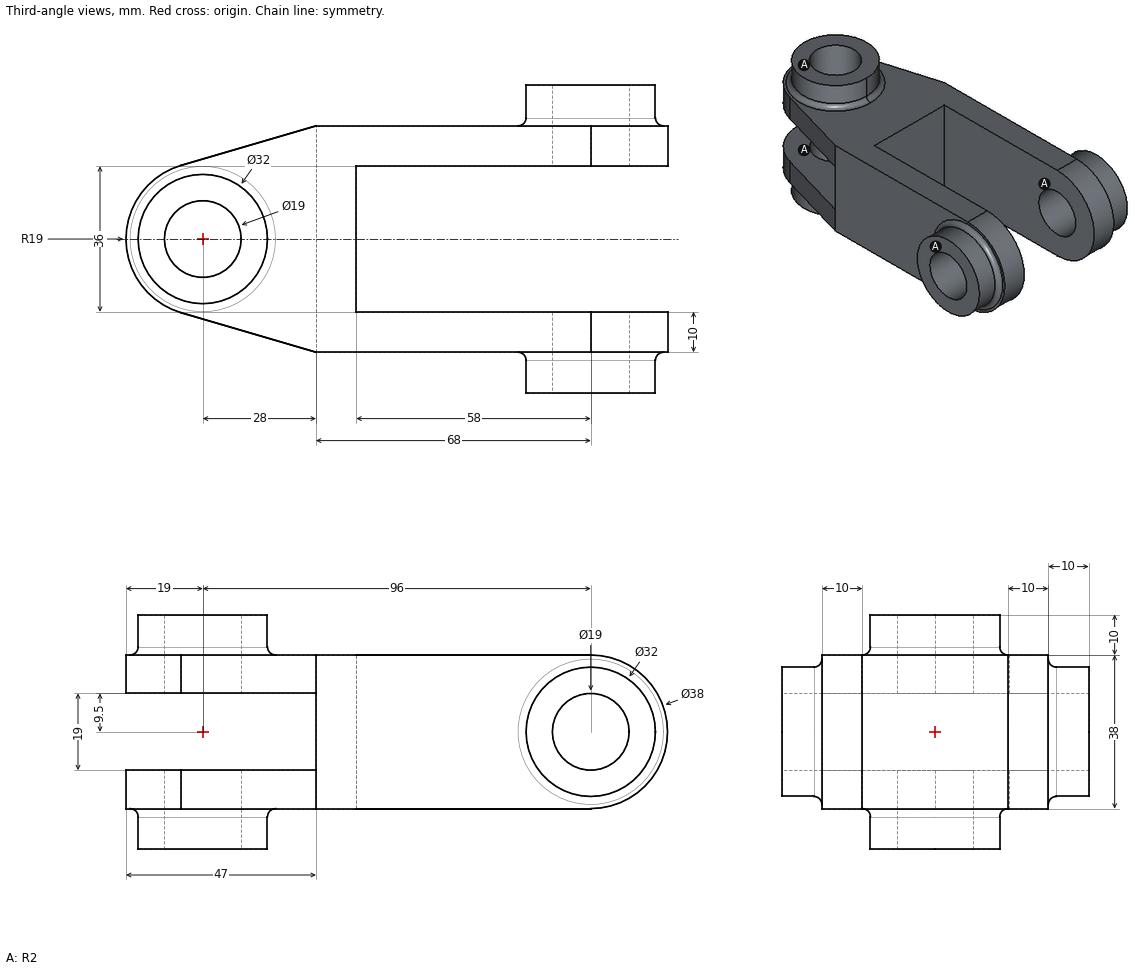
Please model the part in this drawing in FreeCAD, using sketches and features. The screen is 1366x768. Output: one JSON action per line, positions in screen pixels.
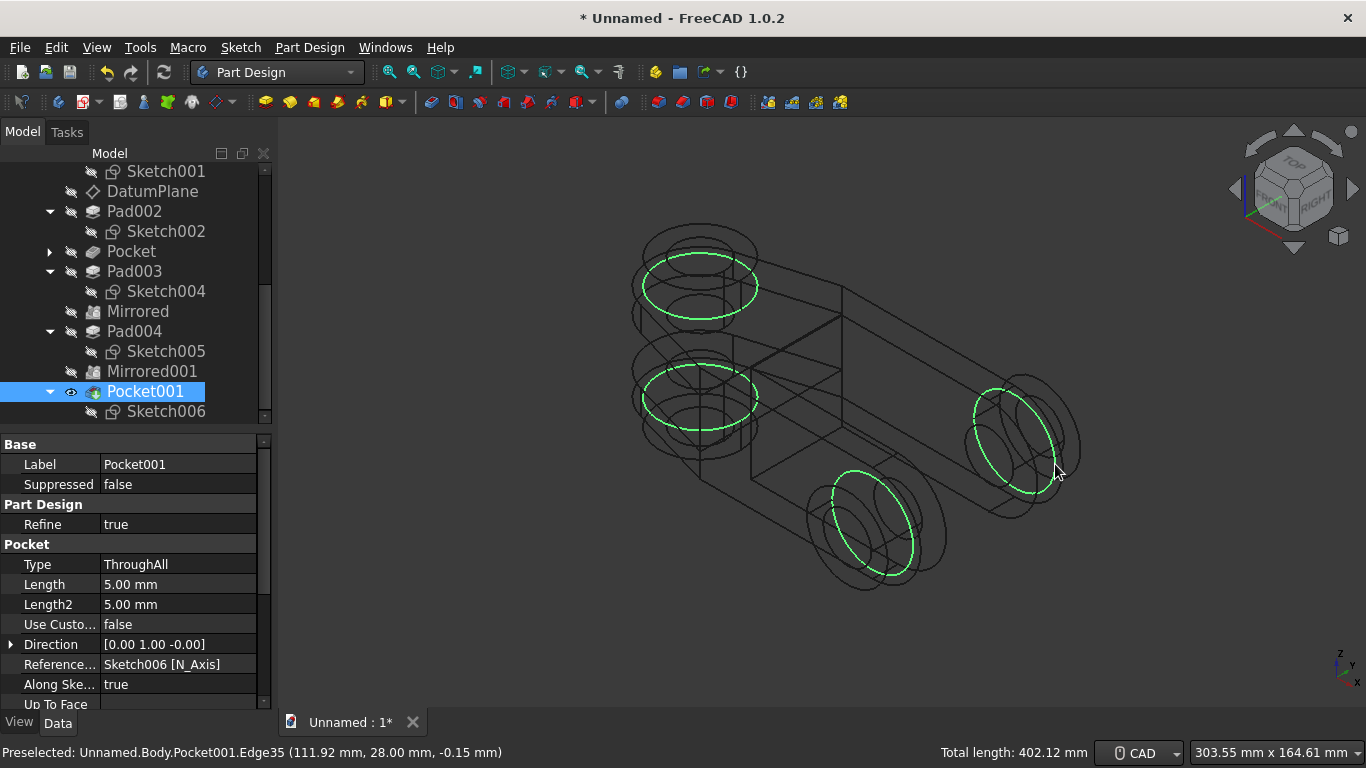
{"action": "key", "text": "v 1"}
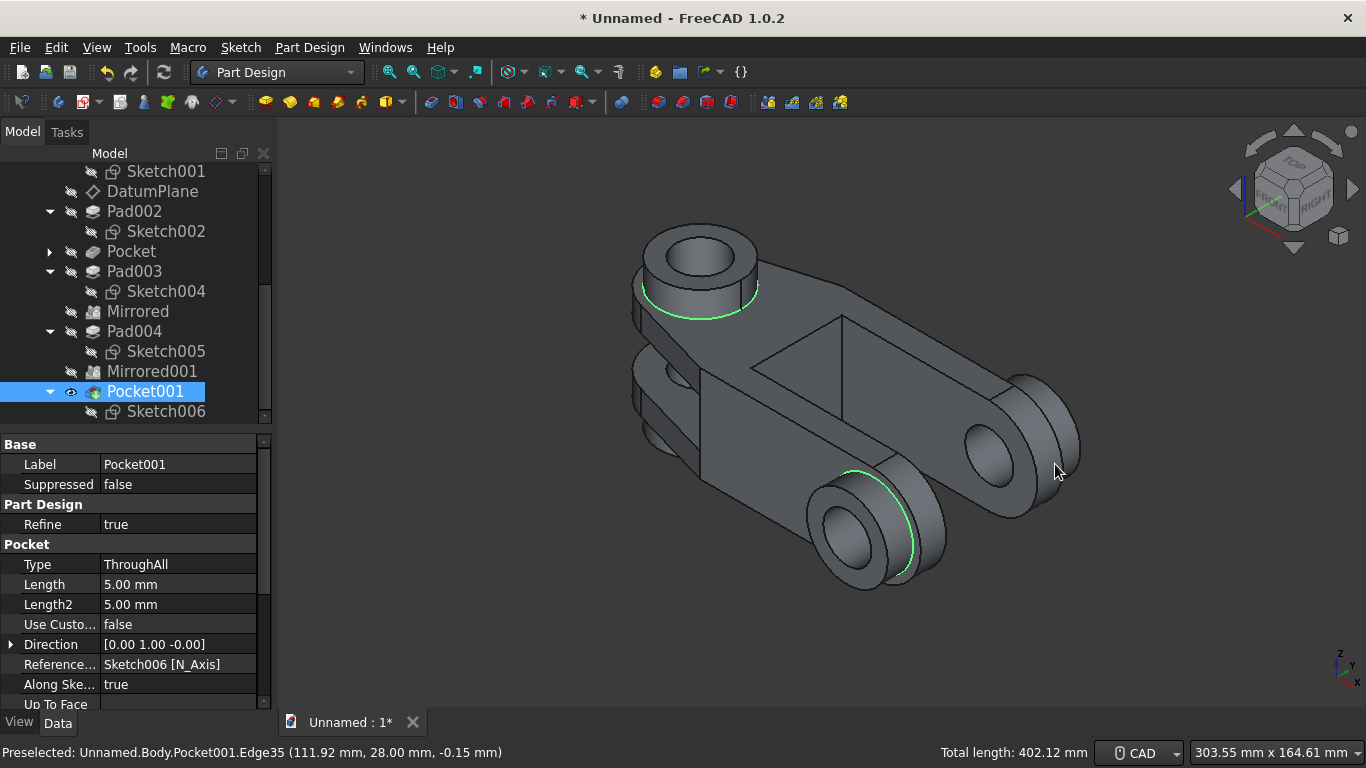
{"action": "left_click", "coordinate": [660, 102]}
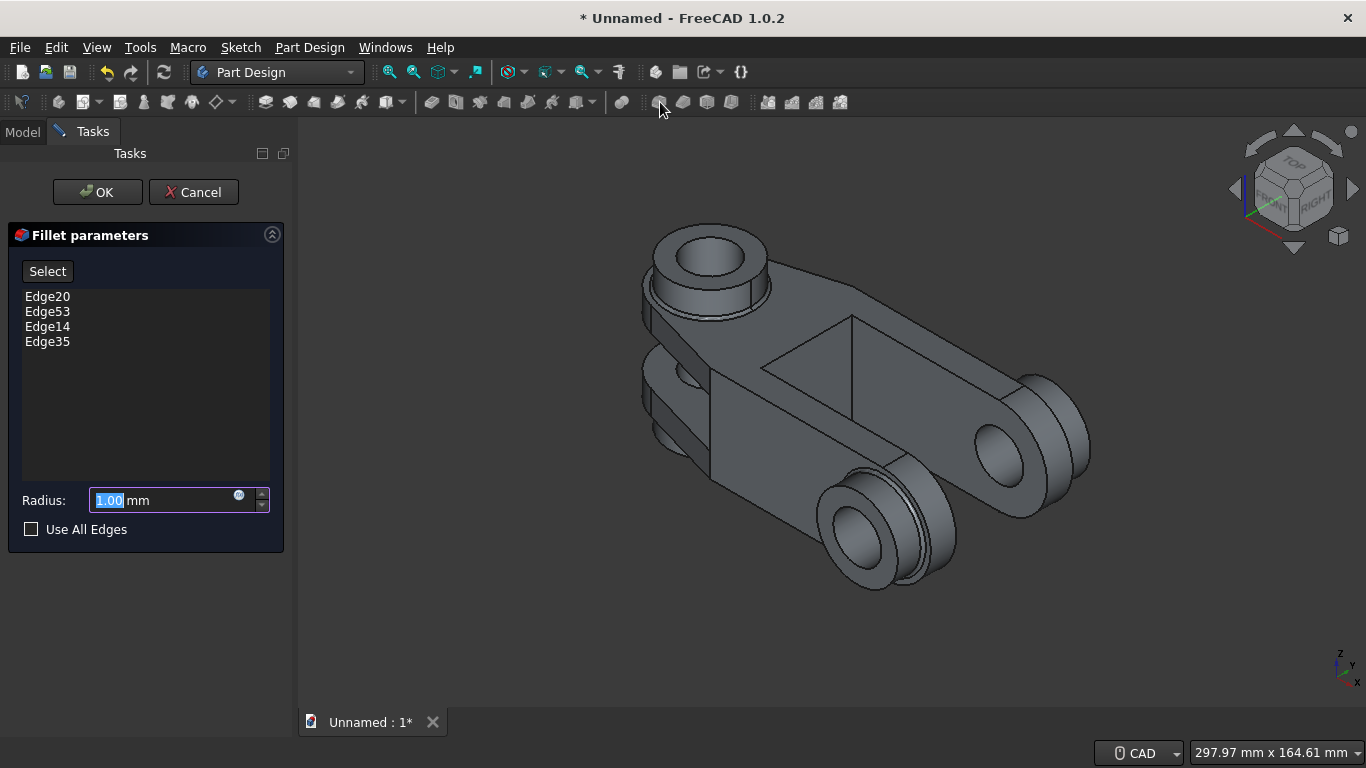
{"action": "type", "text": "2"}
{"action": "key", "text": "Tab"}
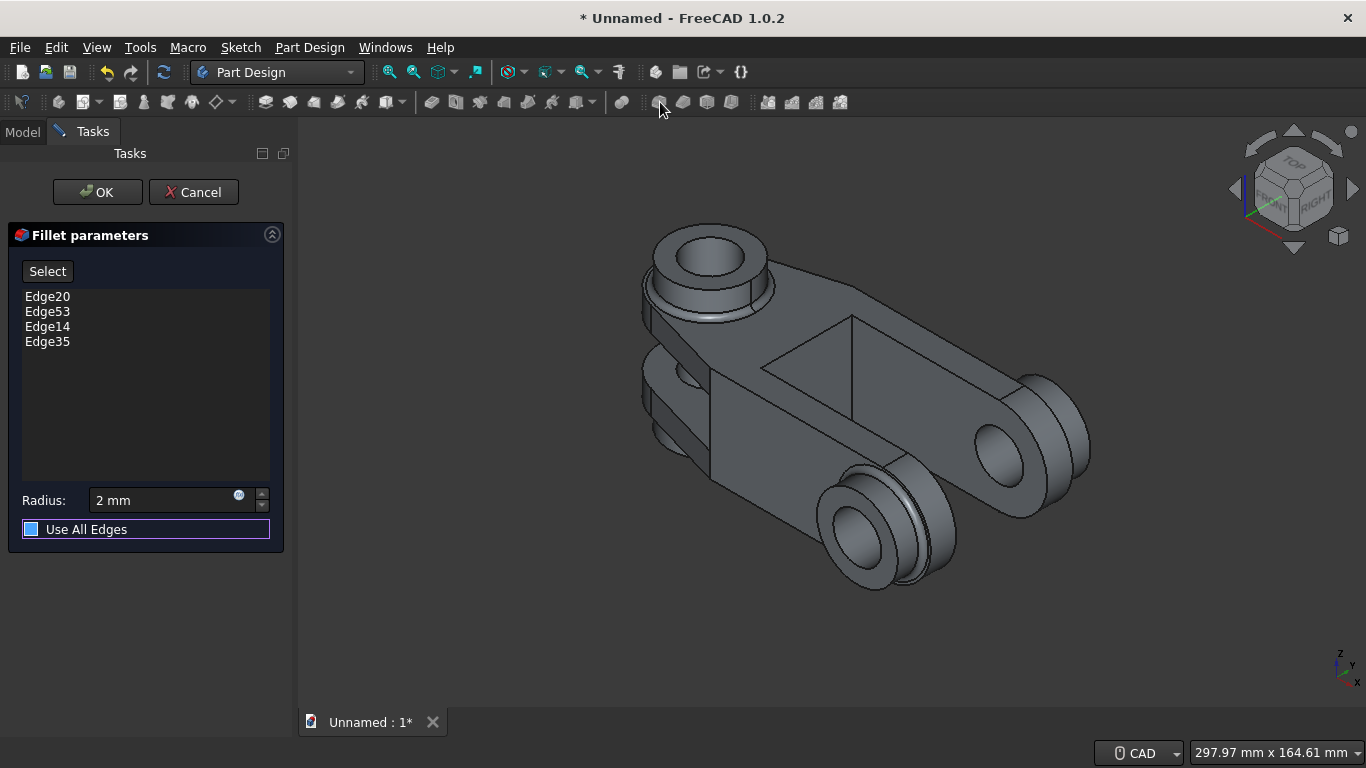
{"action": "left_click", "coordinate": [98, 192]}